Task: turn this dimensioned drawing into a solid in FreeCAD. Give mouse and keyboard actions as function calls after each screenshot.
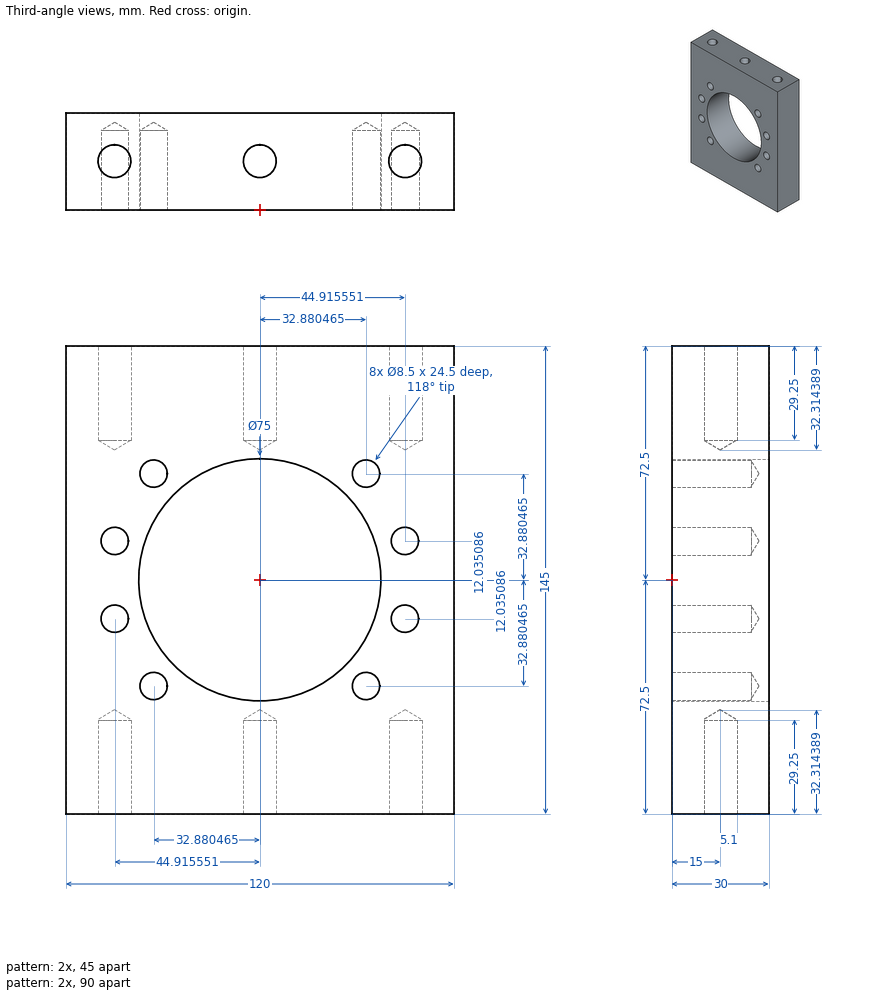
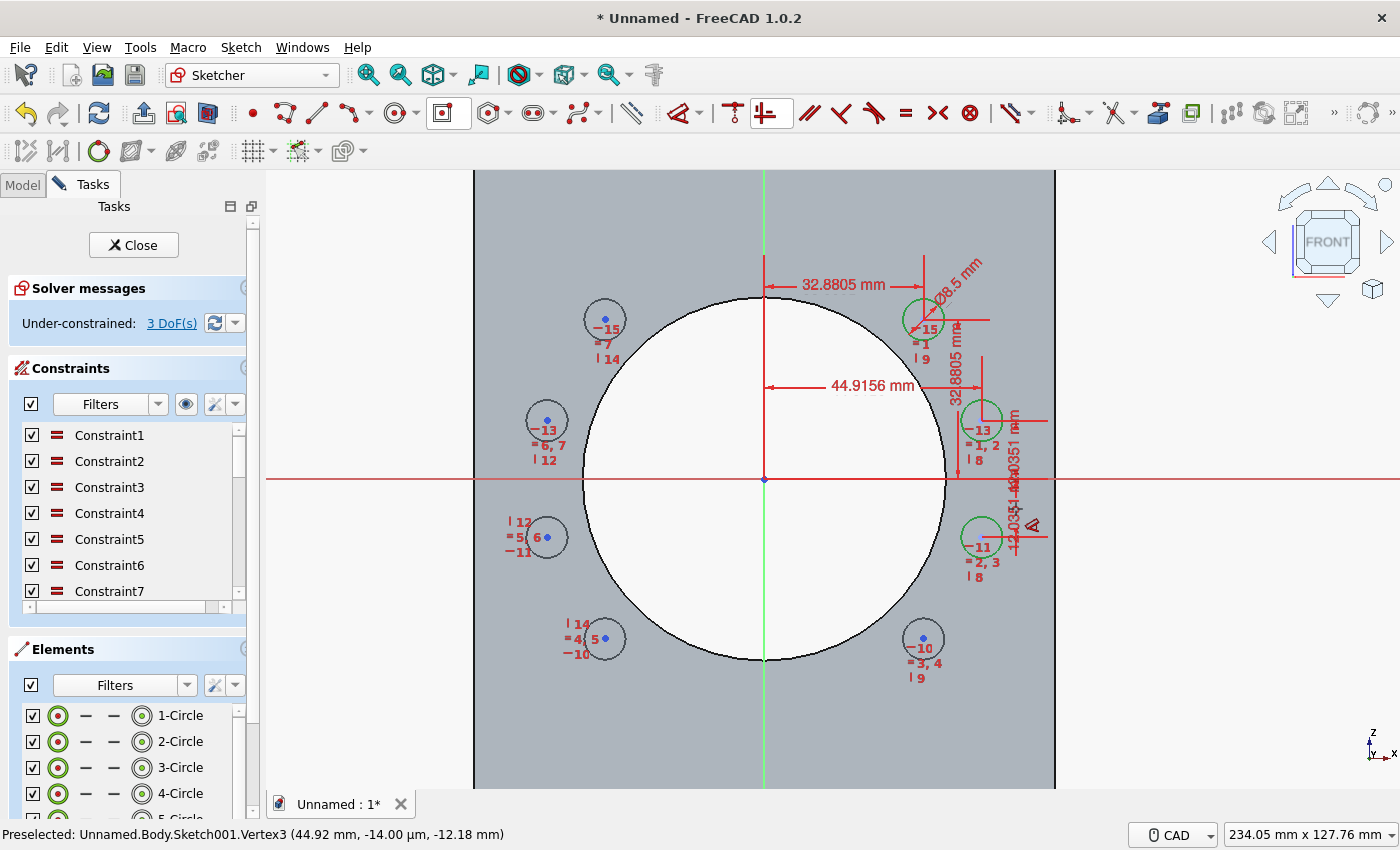
click(924, 639)
click(958, 596)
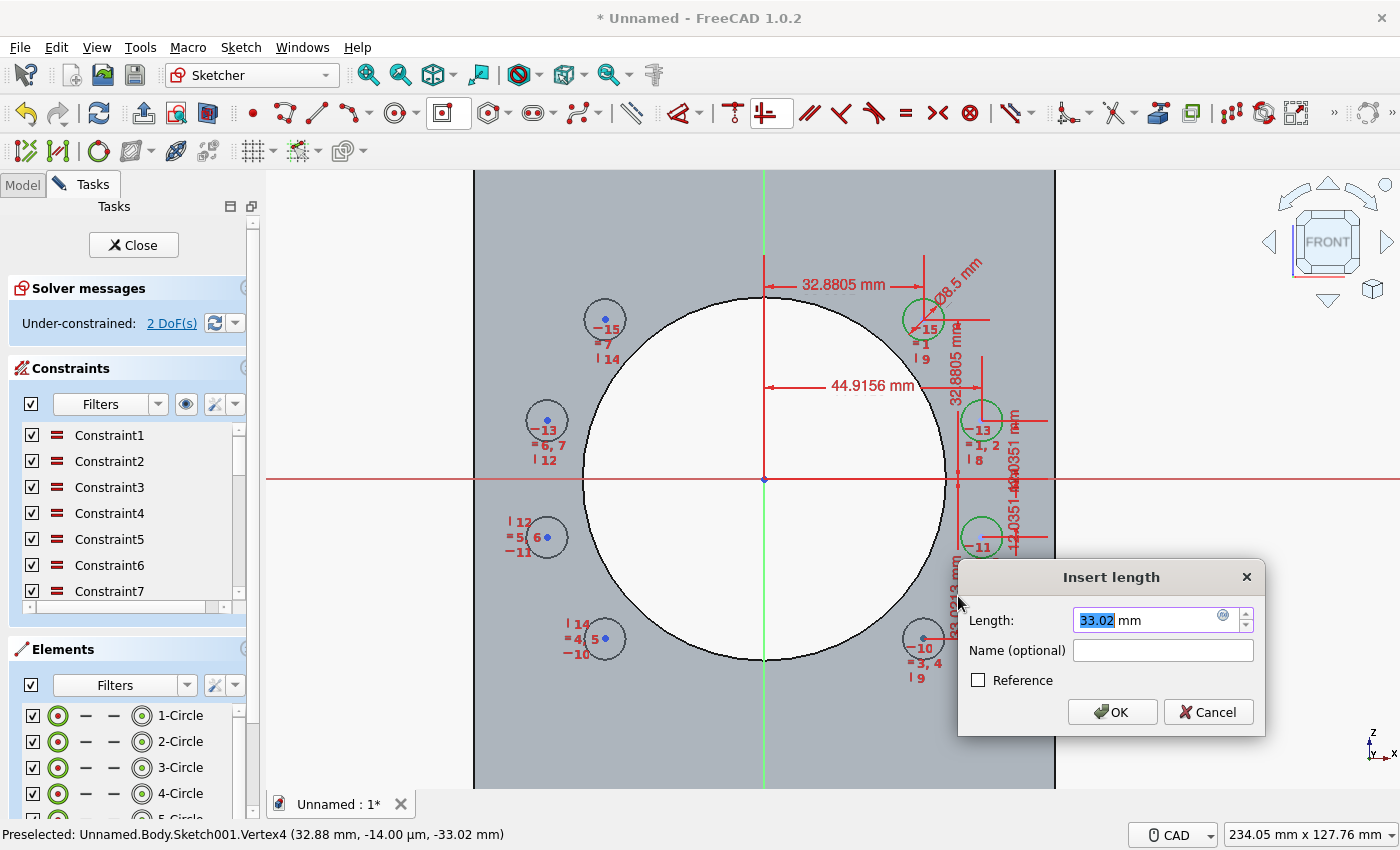
text(32.880465)
key(Return)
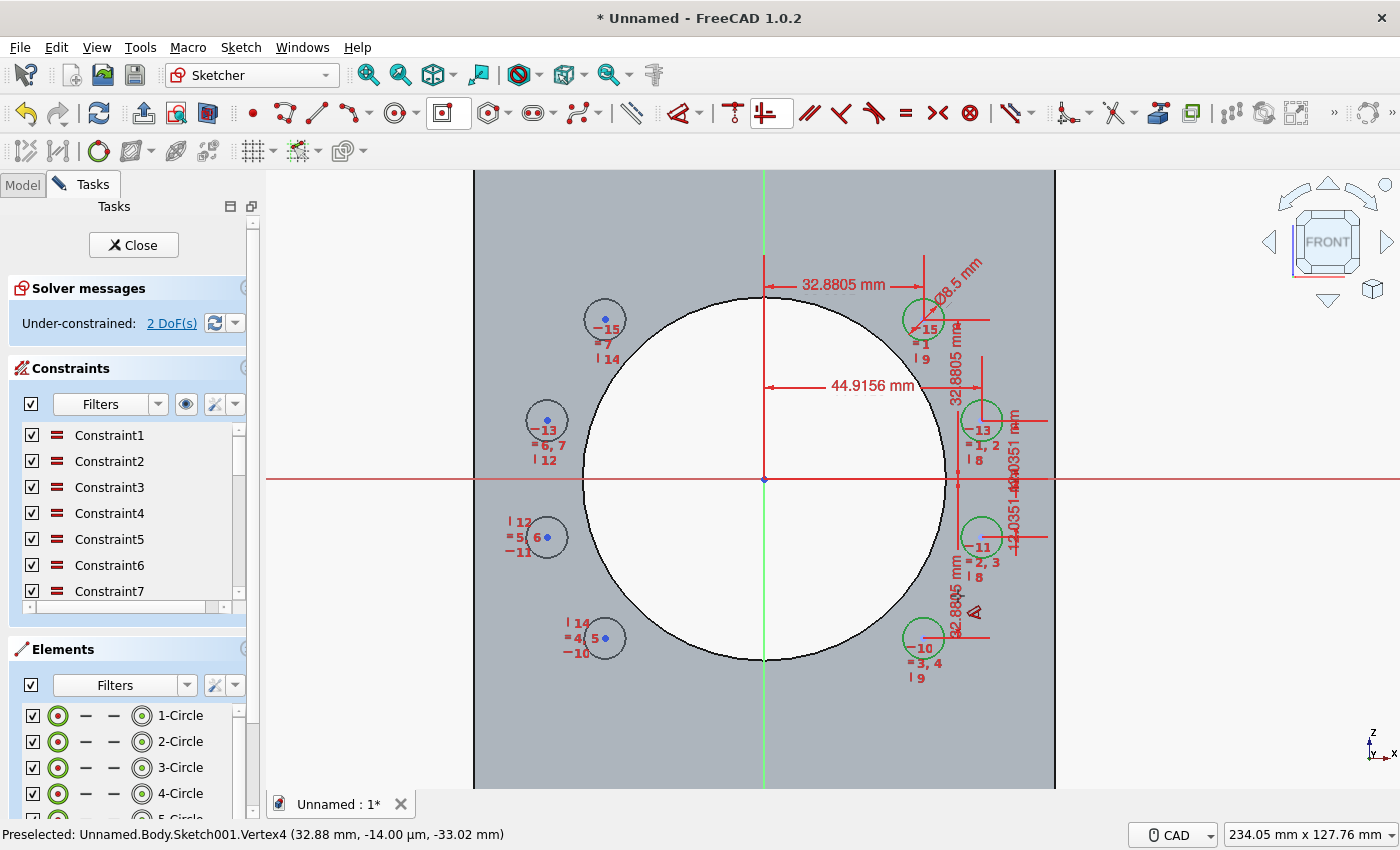
click(605, 638)
click(685, 672)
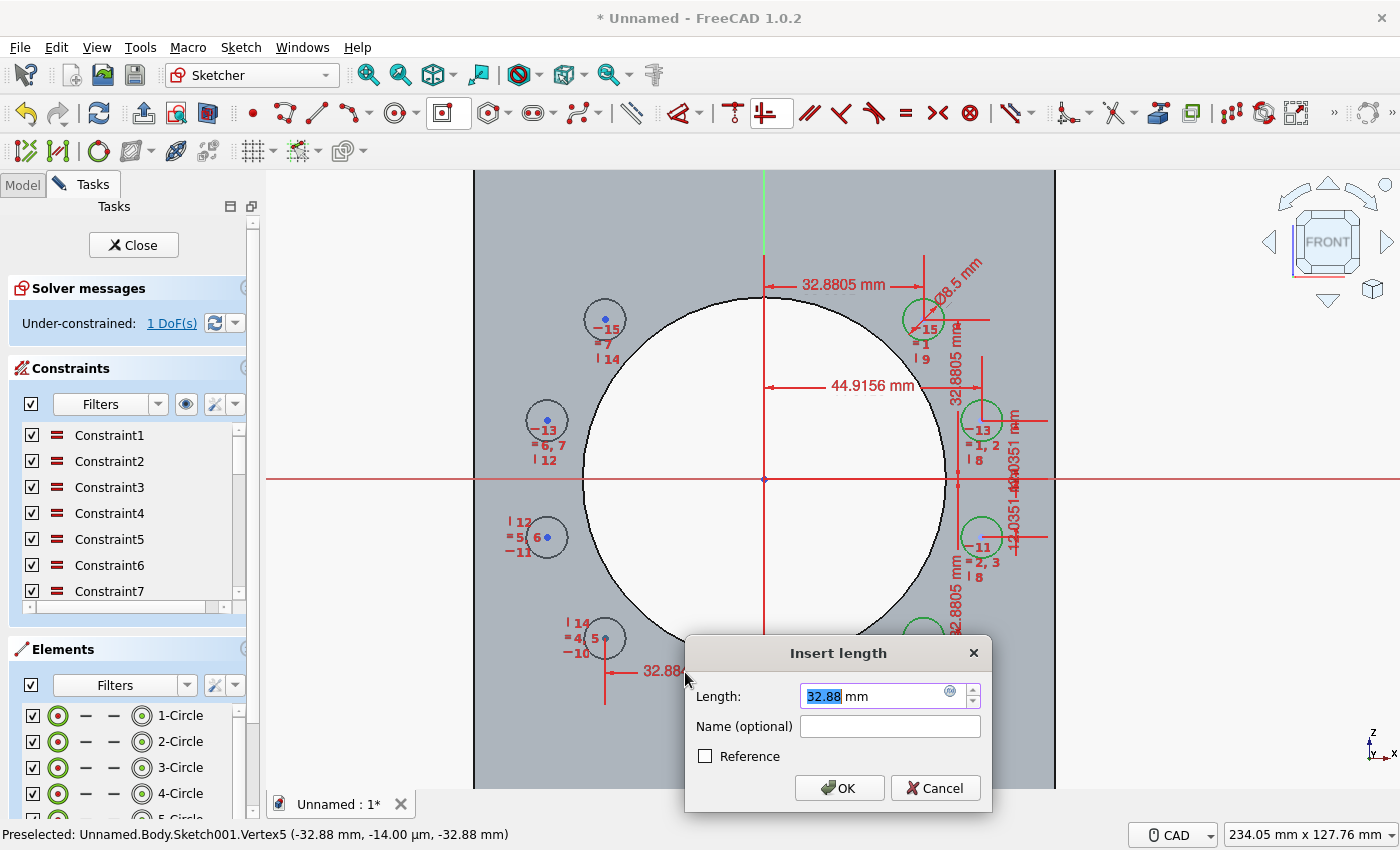
text(32.880465)
key(Return)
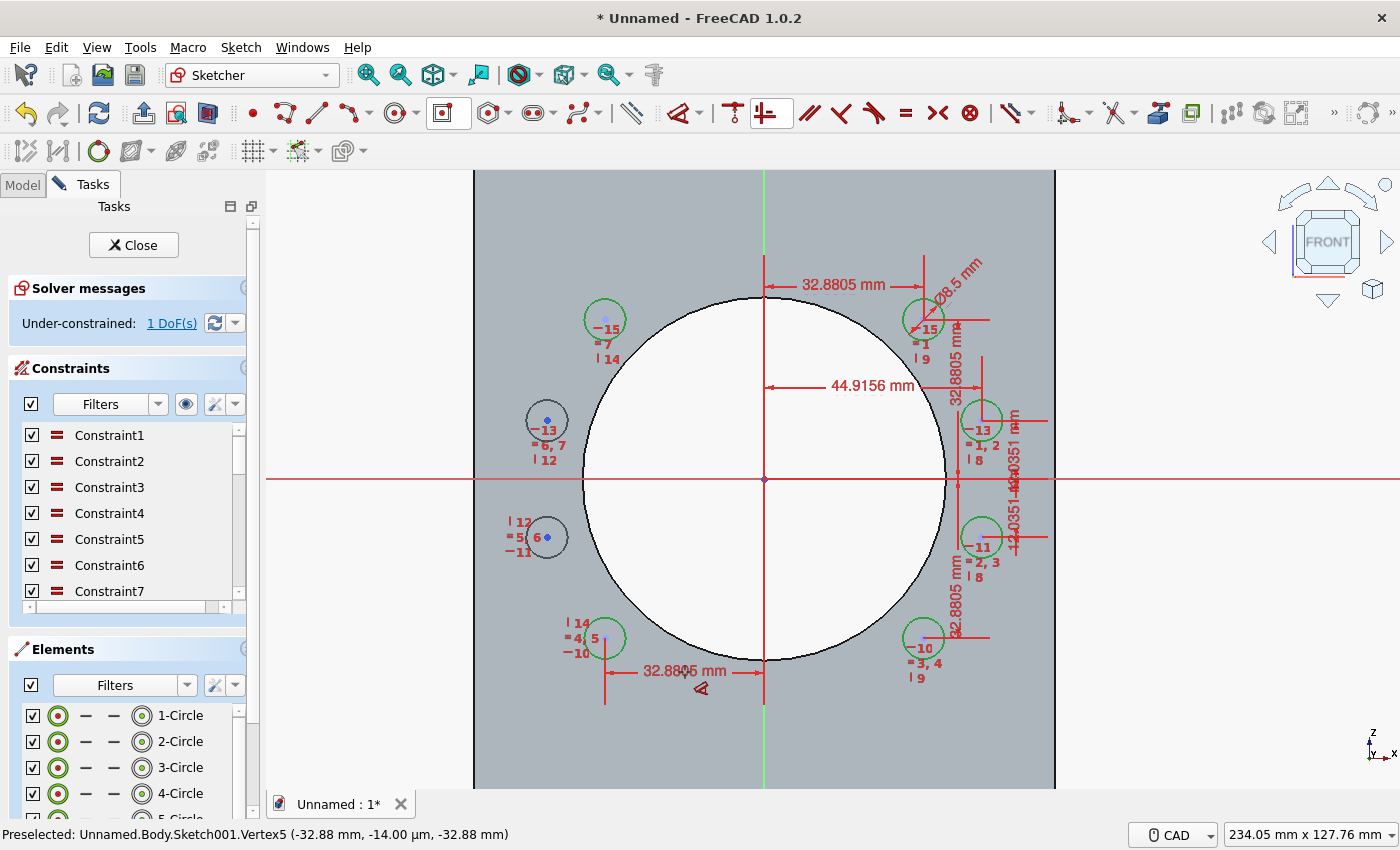
click(547, 537)
click(656, 571)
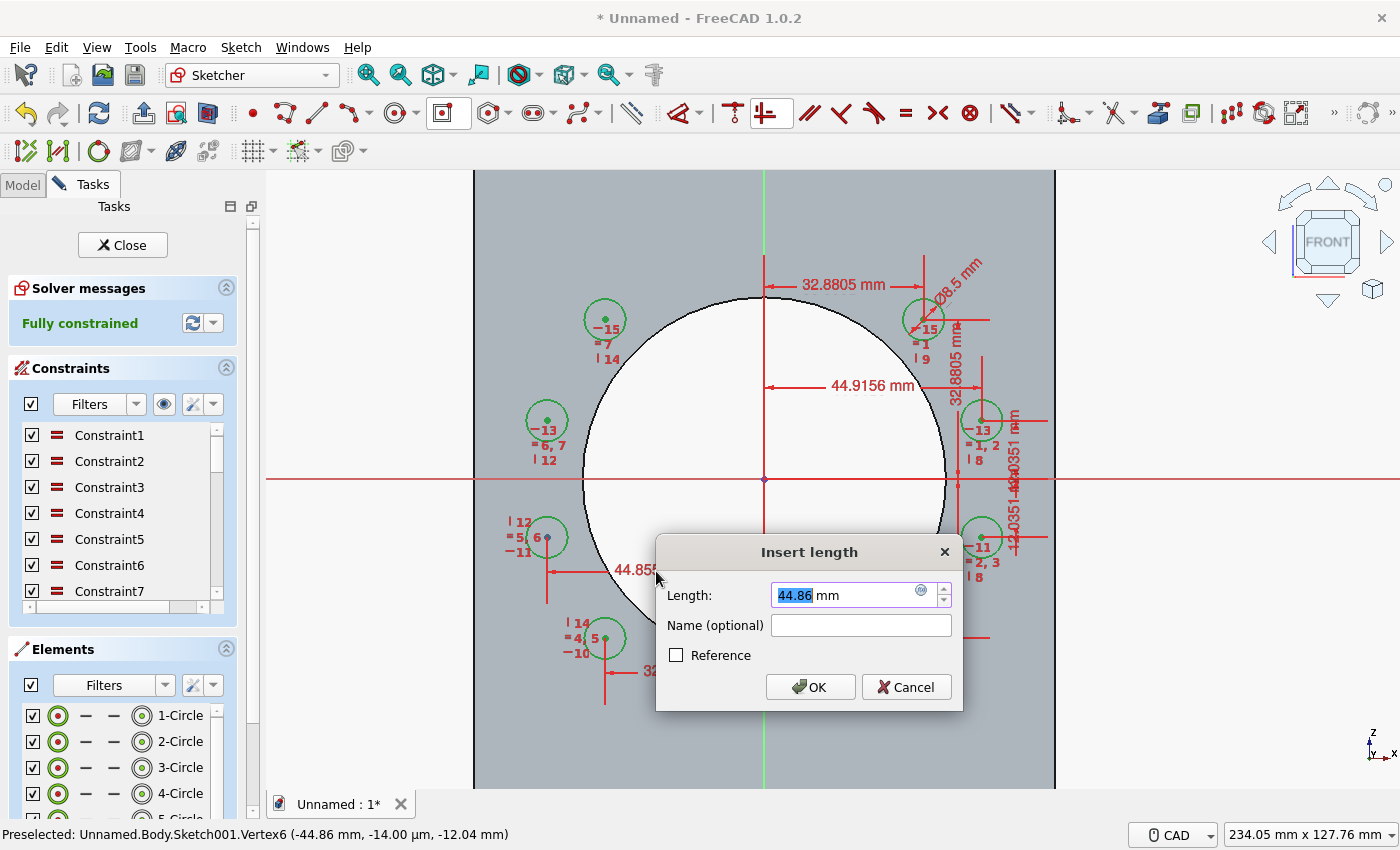
text(44.915551)
key(Return)
key(Escape)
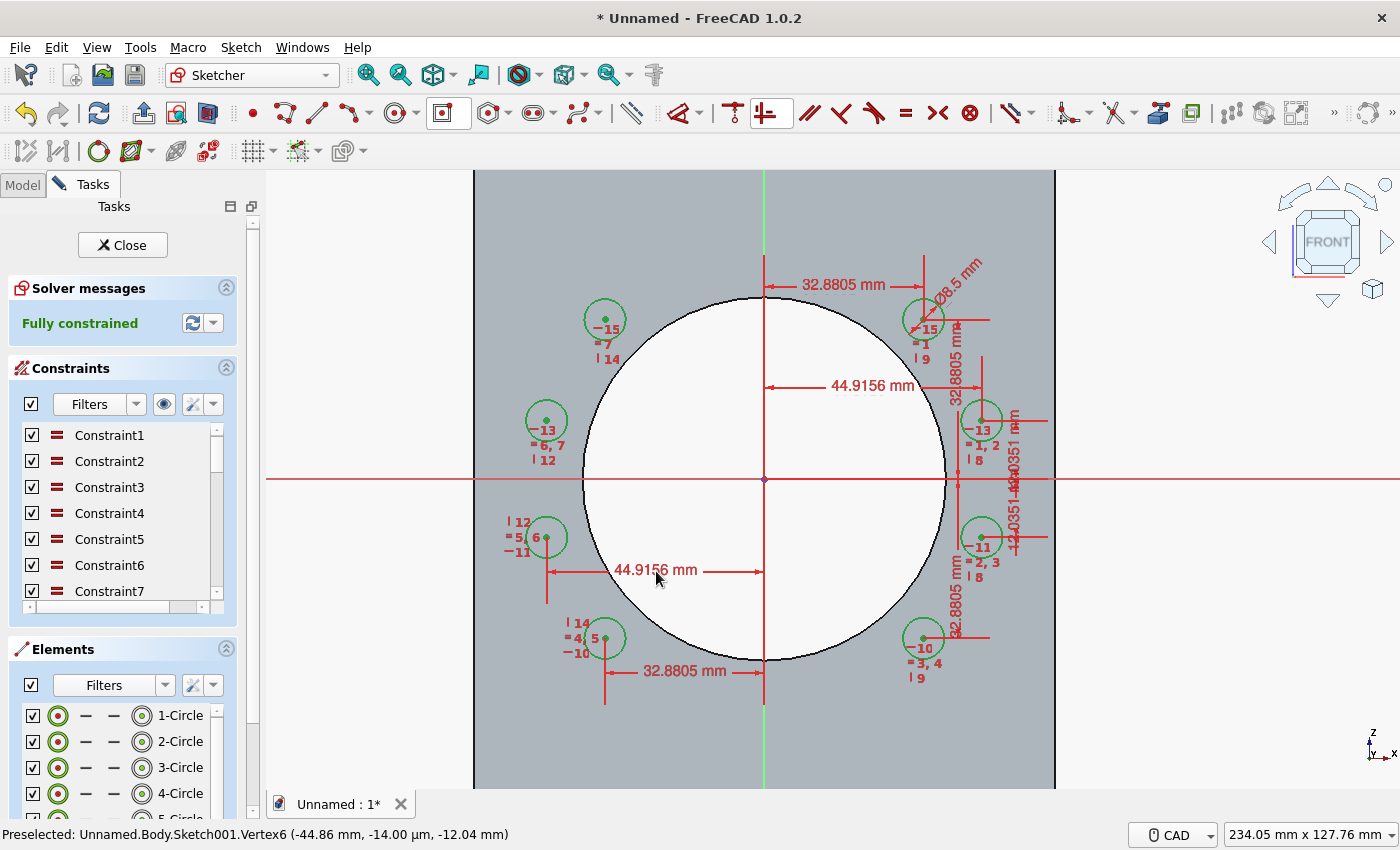
click(123, 245)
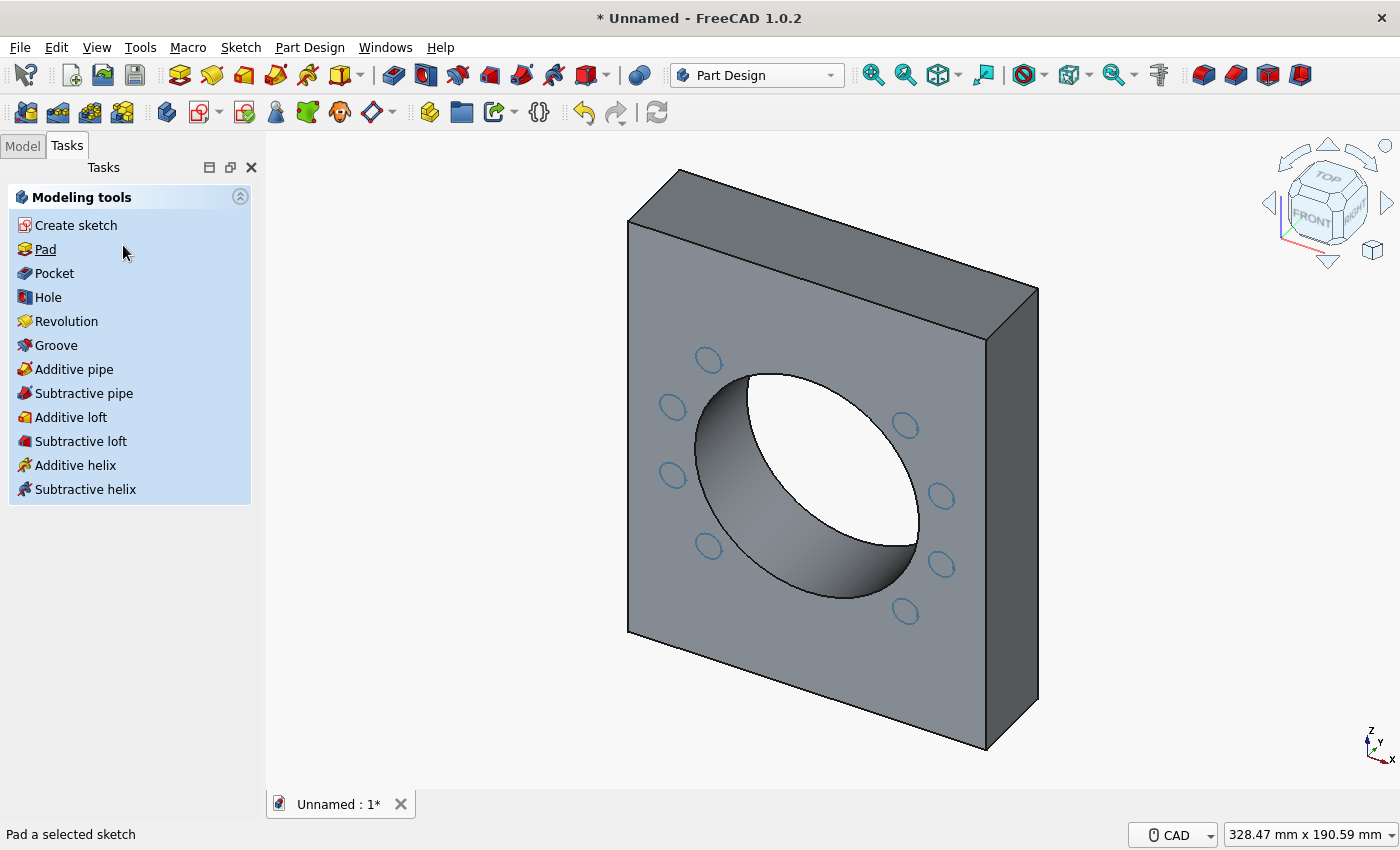
click(426, 76)